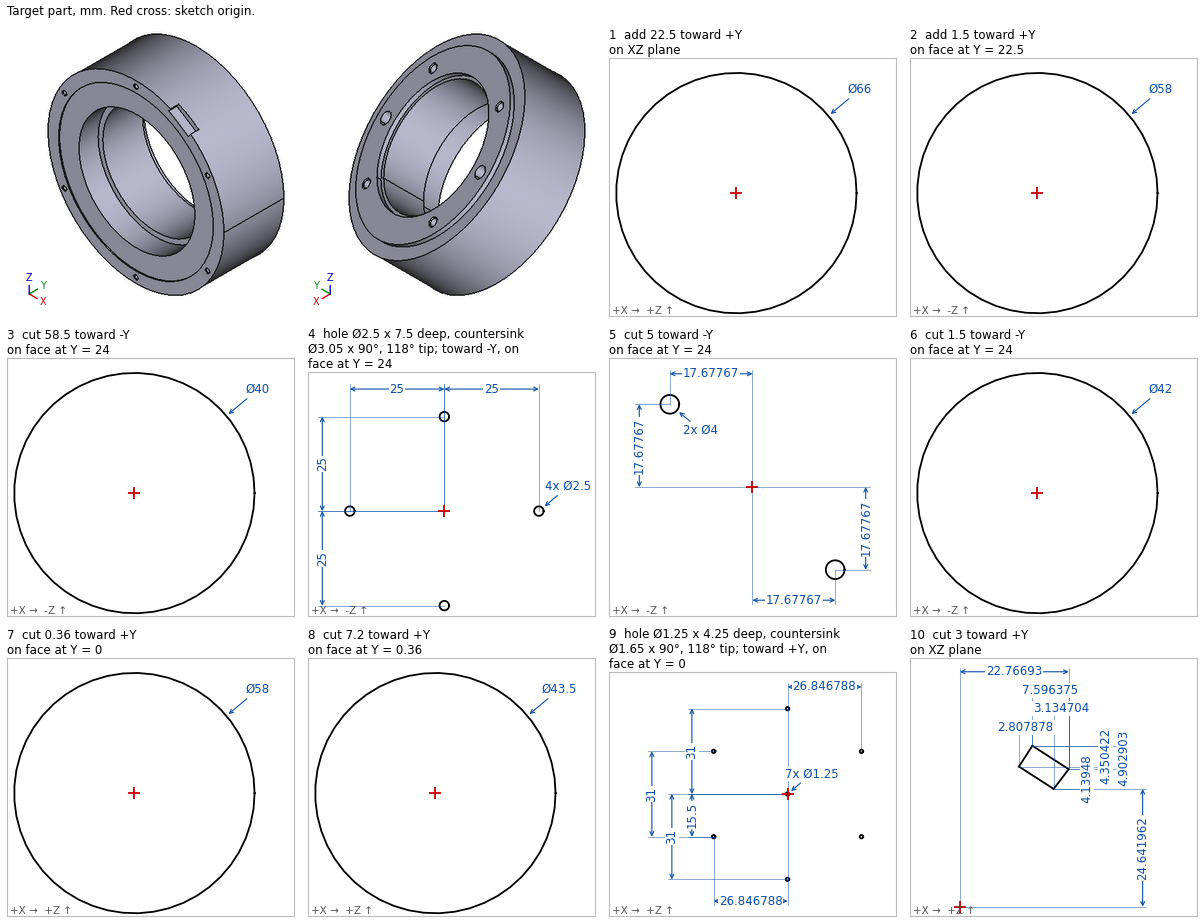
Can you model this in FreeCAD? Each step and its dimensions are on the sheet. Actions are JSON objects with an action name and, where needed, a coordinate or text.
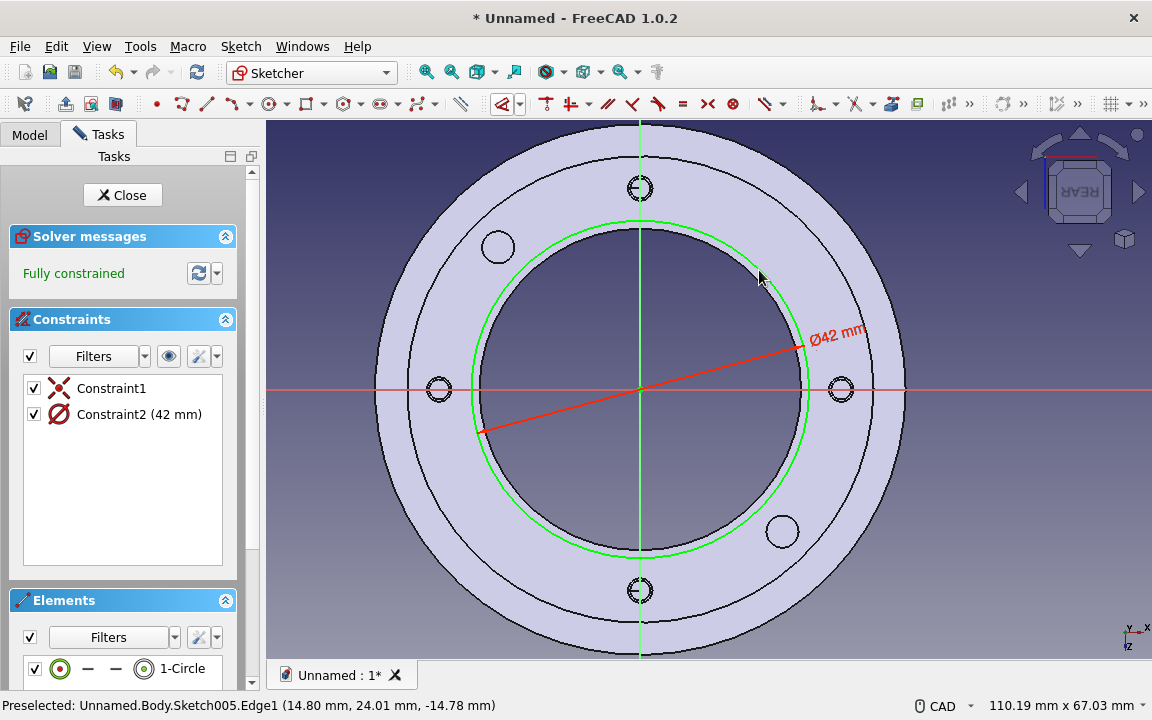
{"action": "left_click", "coordinate": [123, 195]}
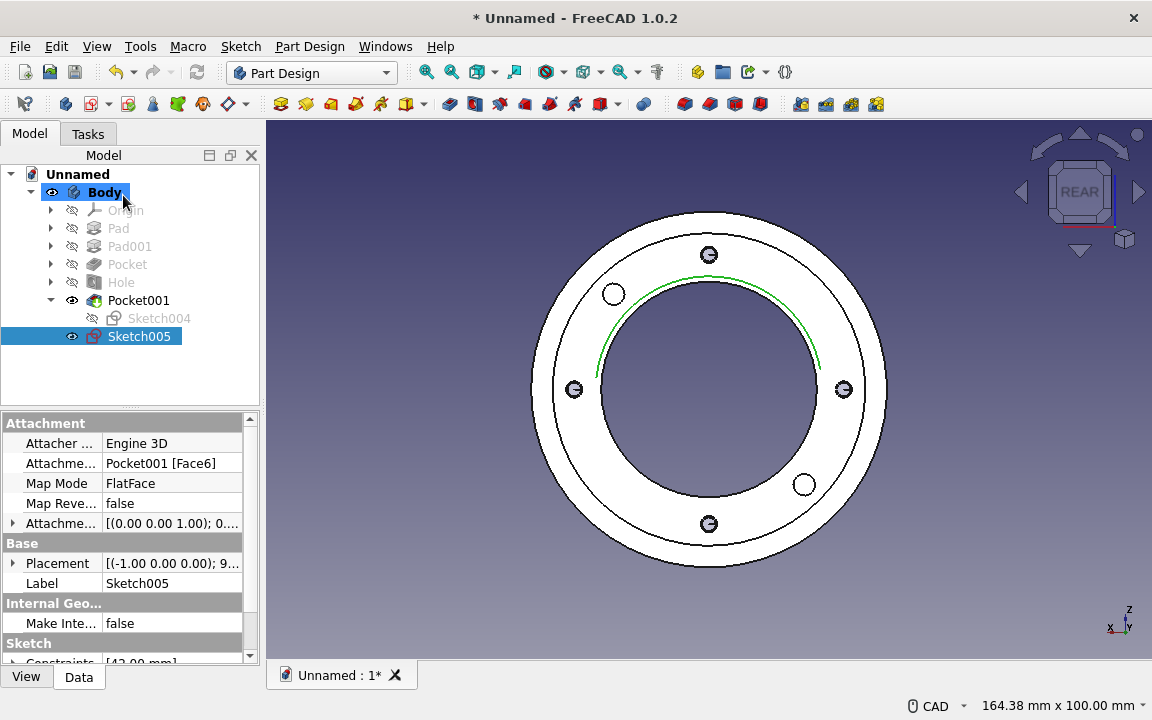
{"action": "left_click", "coordinate": [450, 104]}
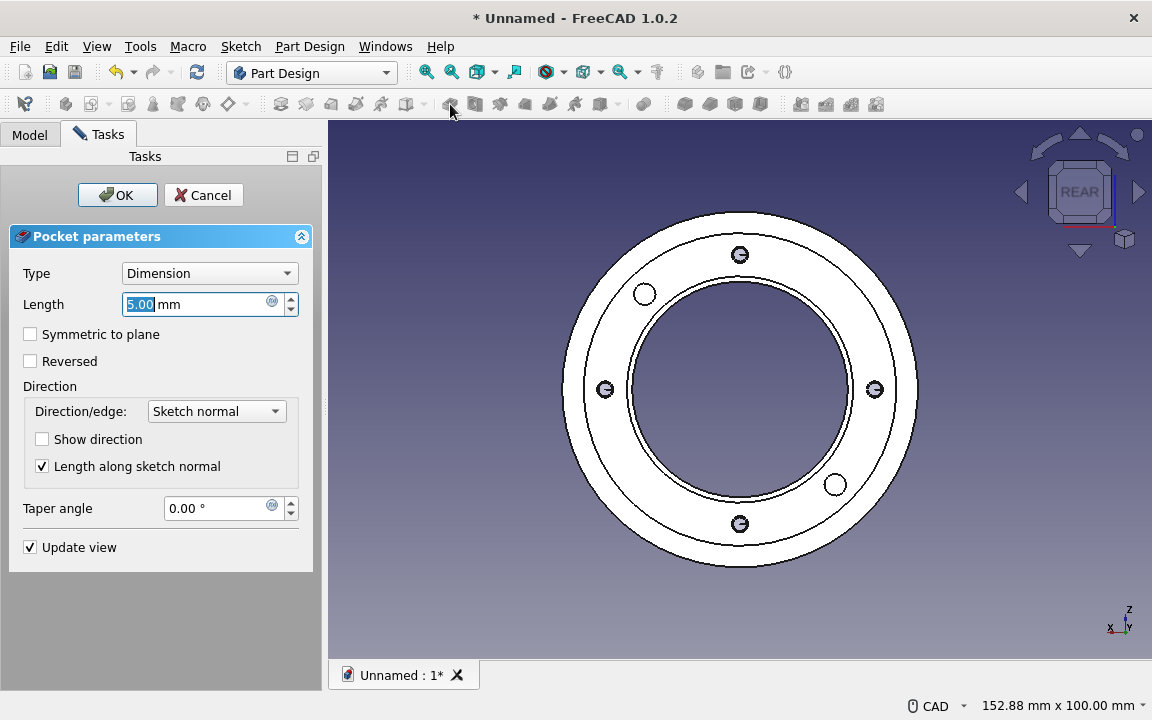
{"action": "type", "text": "1.5"}
{"action": "key", "text": "Tab"}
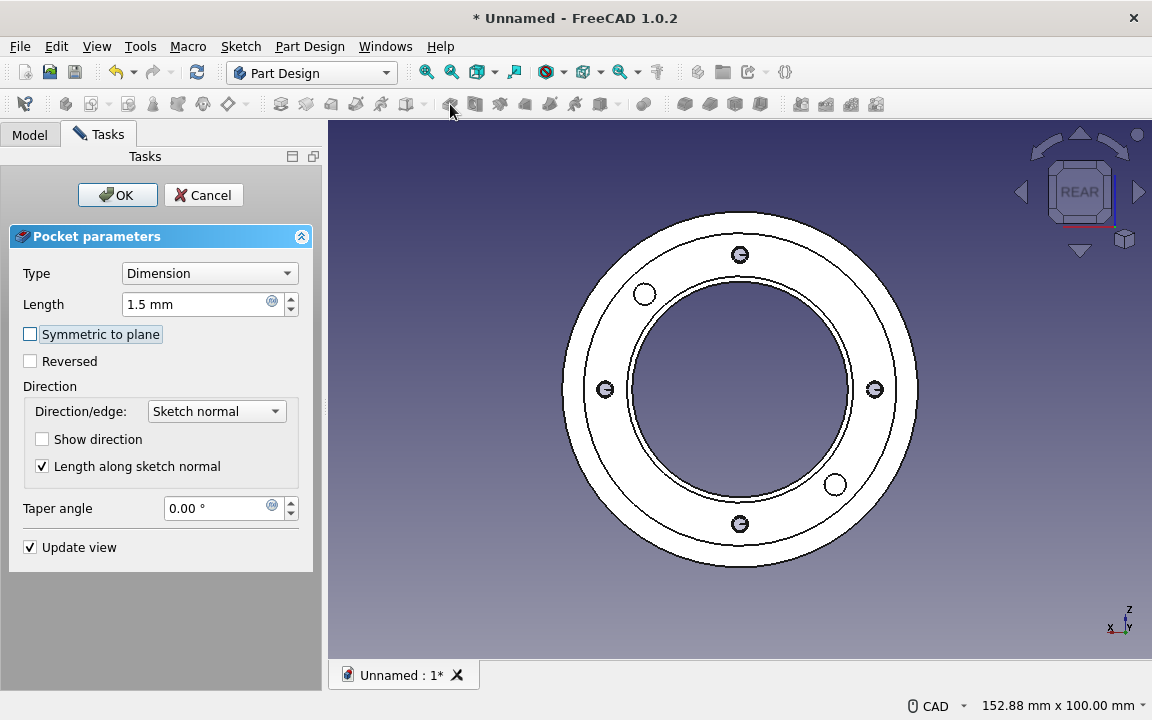
{"action": "left_click", "coordinate": [118, 195]}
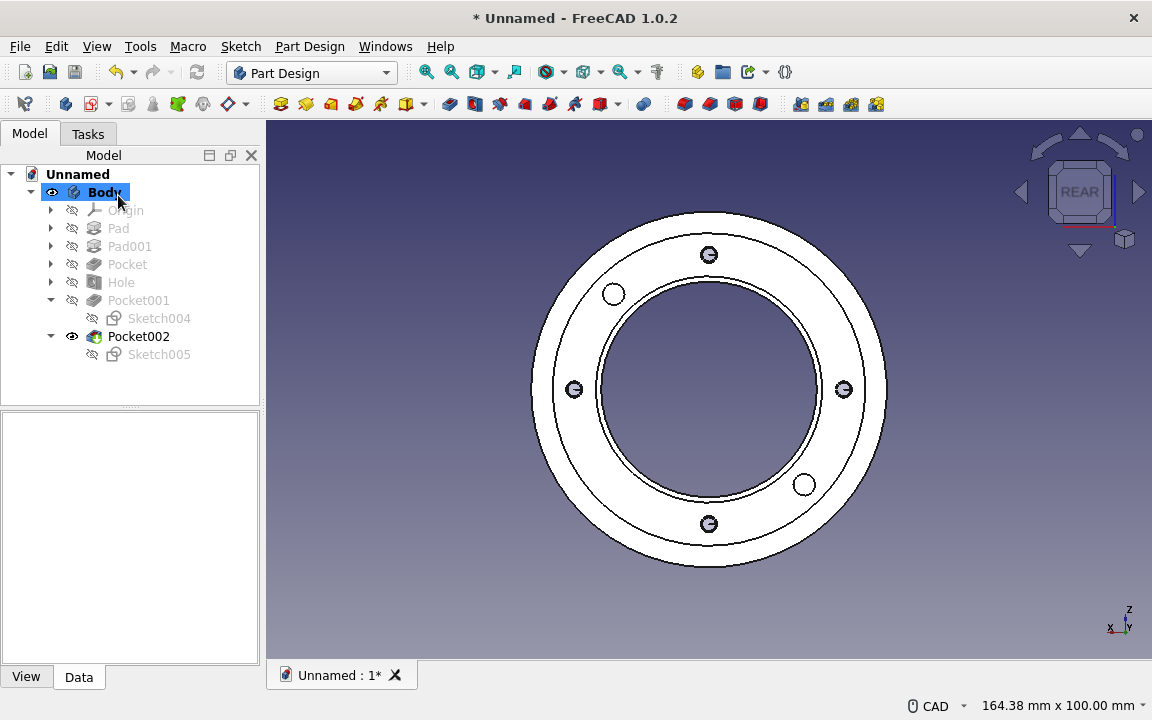
{"action": "key", "text": "0"}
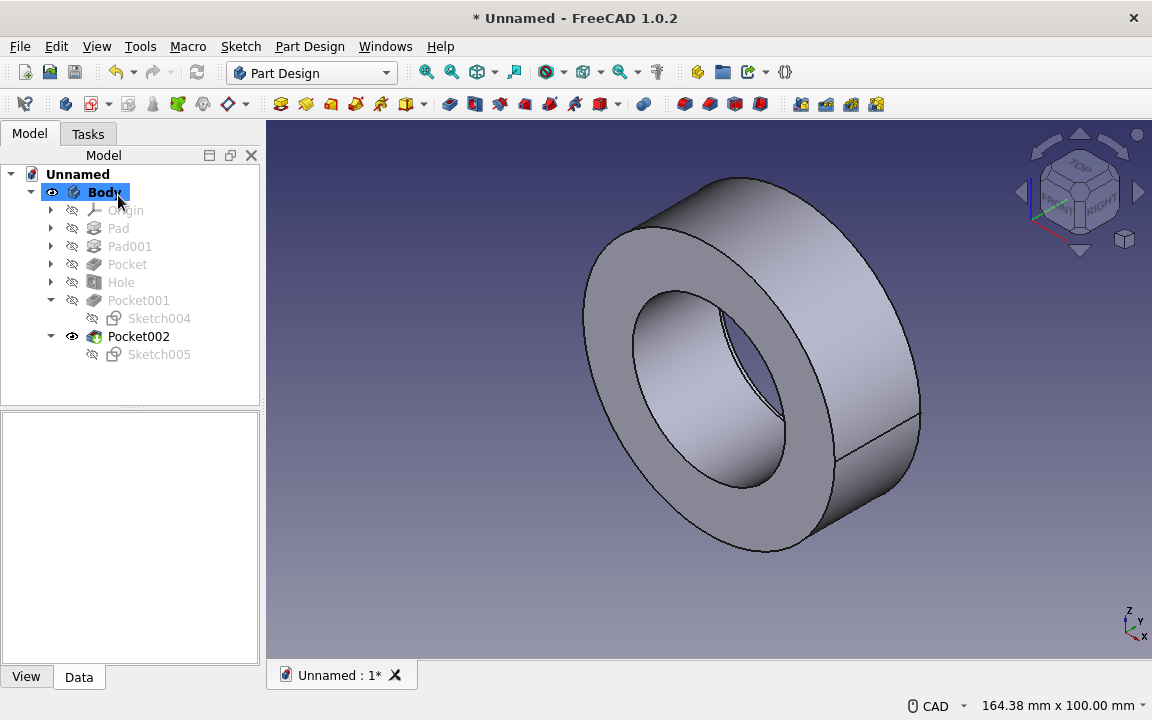
{"action": "left_click", "coordinate": [427, 72]}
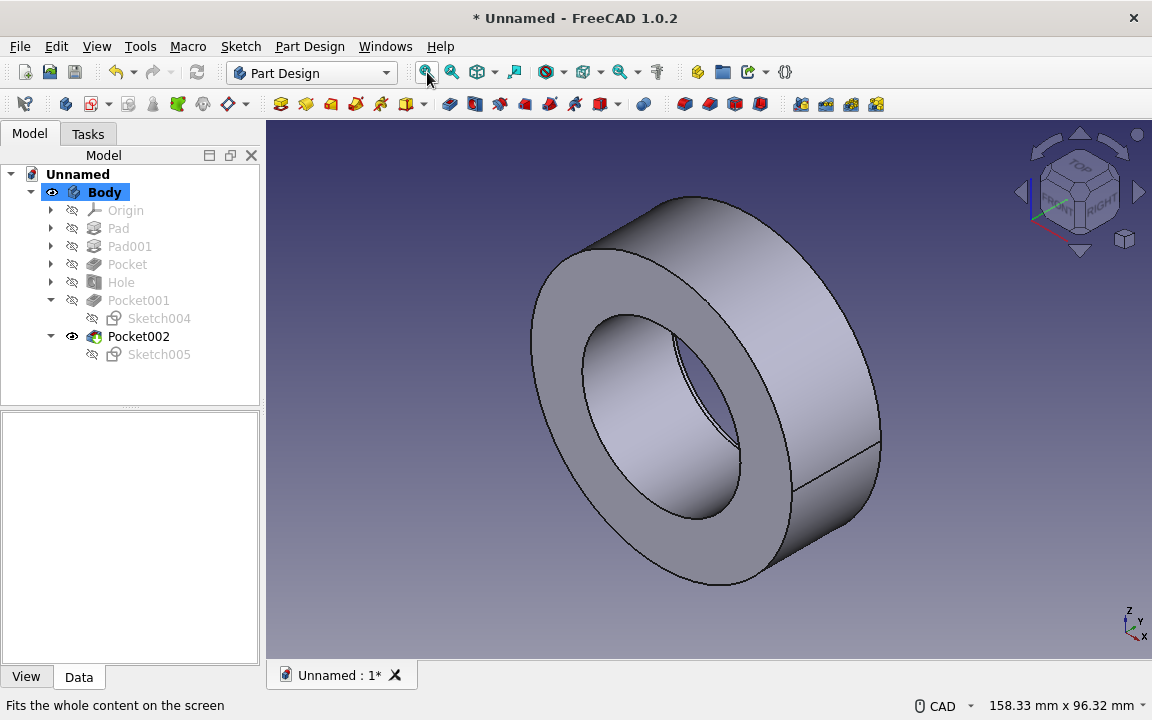
{"action": "left_click", "coordinate": [736, 373]}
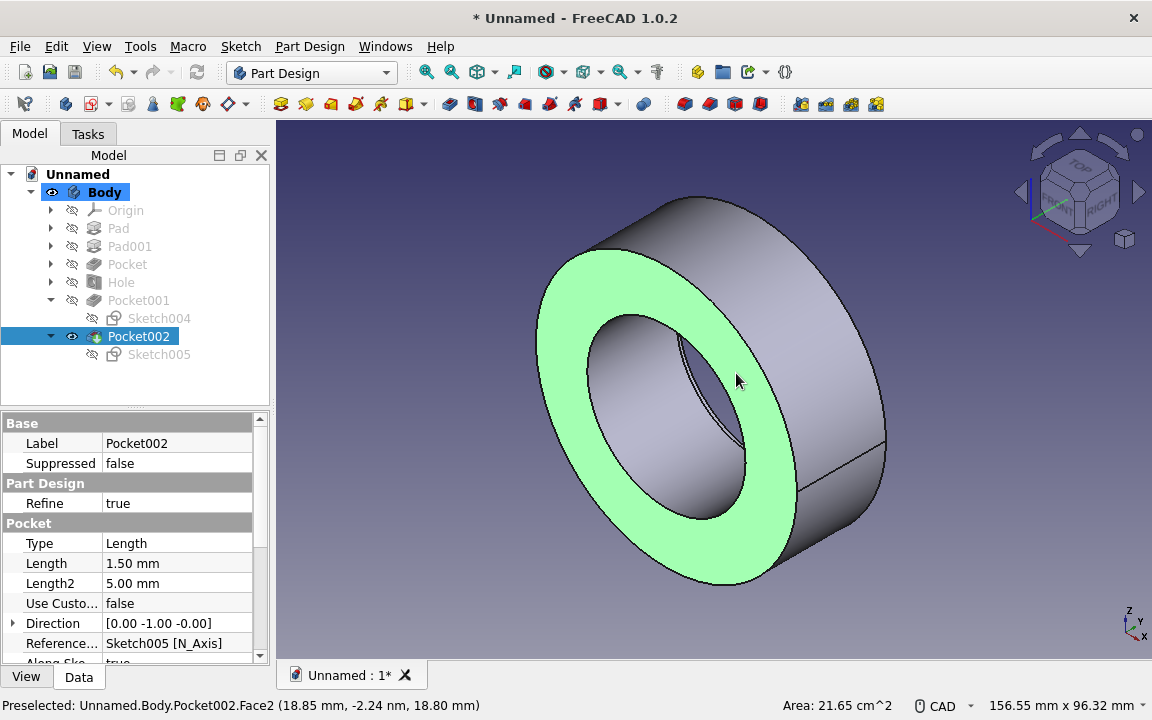
{"action": "left_click", "coordinate": [90, 104]}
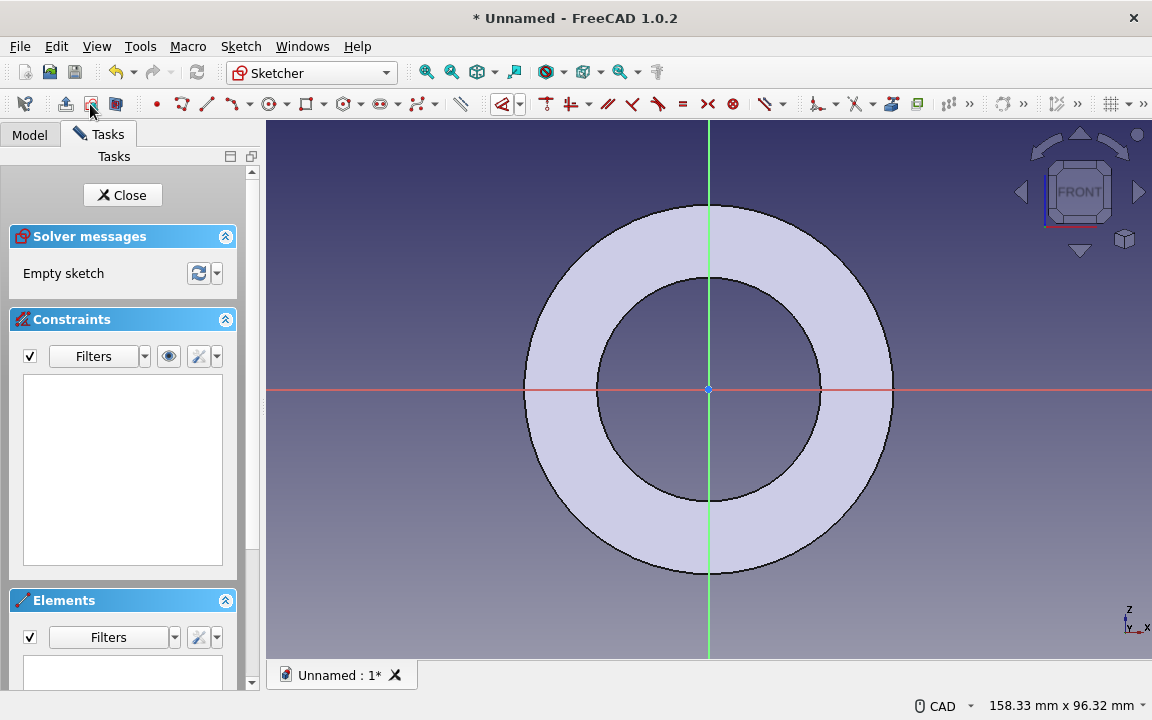
{"action": "left_click", "coordinate": [268, 104]}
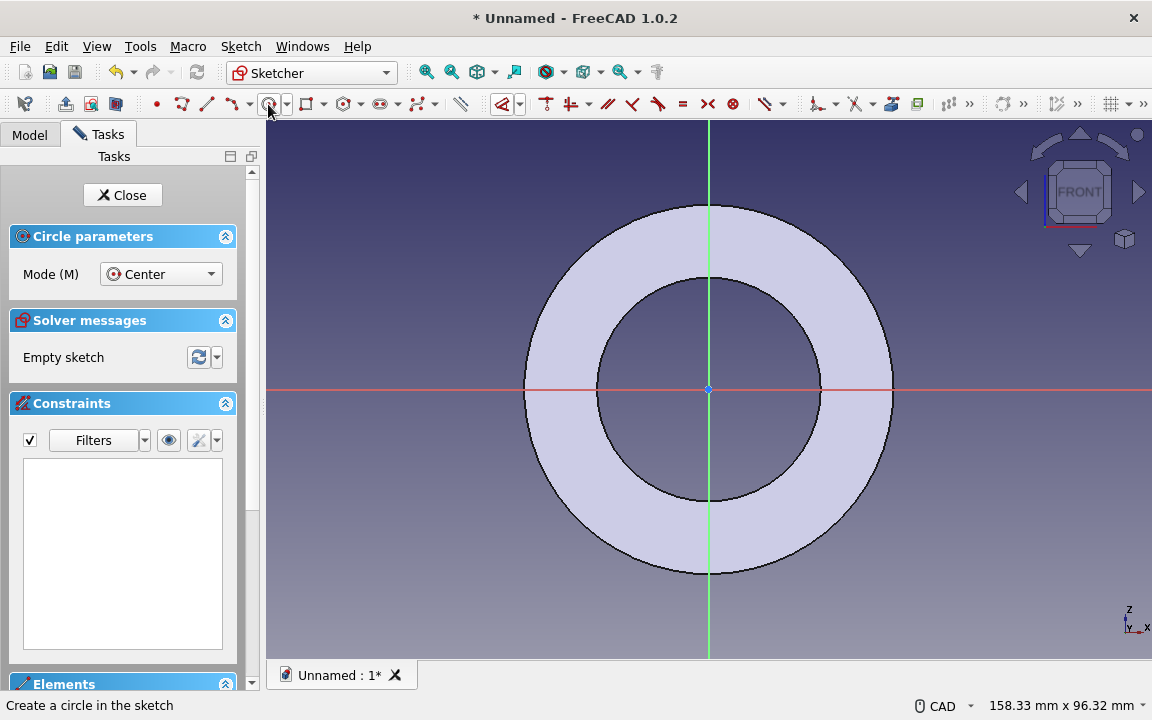
{"action": "left_click", "coordinate": [709, 390]}
{"action": "left_click", "coordinate": [824, 275]}
{"action": "key", "text": "Escape"}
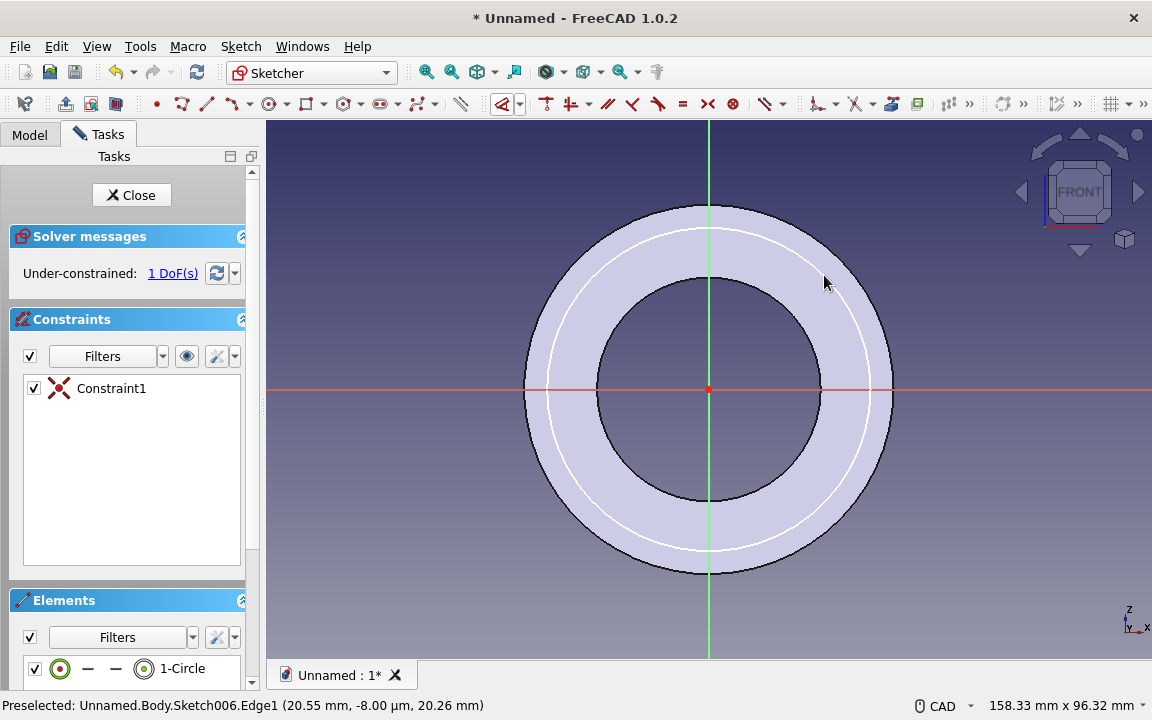
{"action": "left_click", "coordinate": [823, 275]}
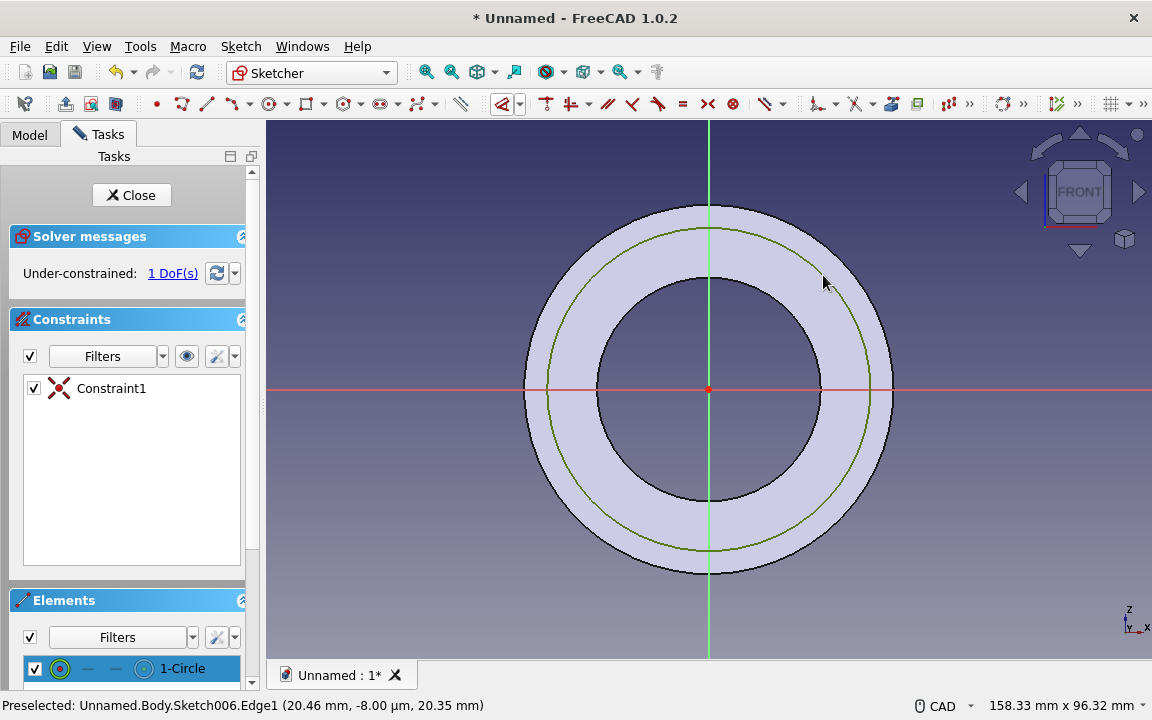
{"action": "left_click", "coordinate": [520, 104]}